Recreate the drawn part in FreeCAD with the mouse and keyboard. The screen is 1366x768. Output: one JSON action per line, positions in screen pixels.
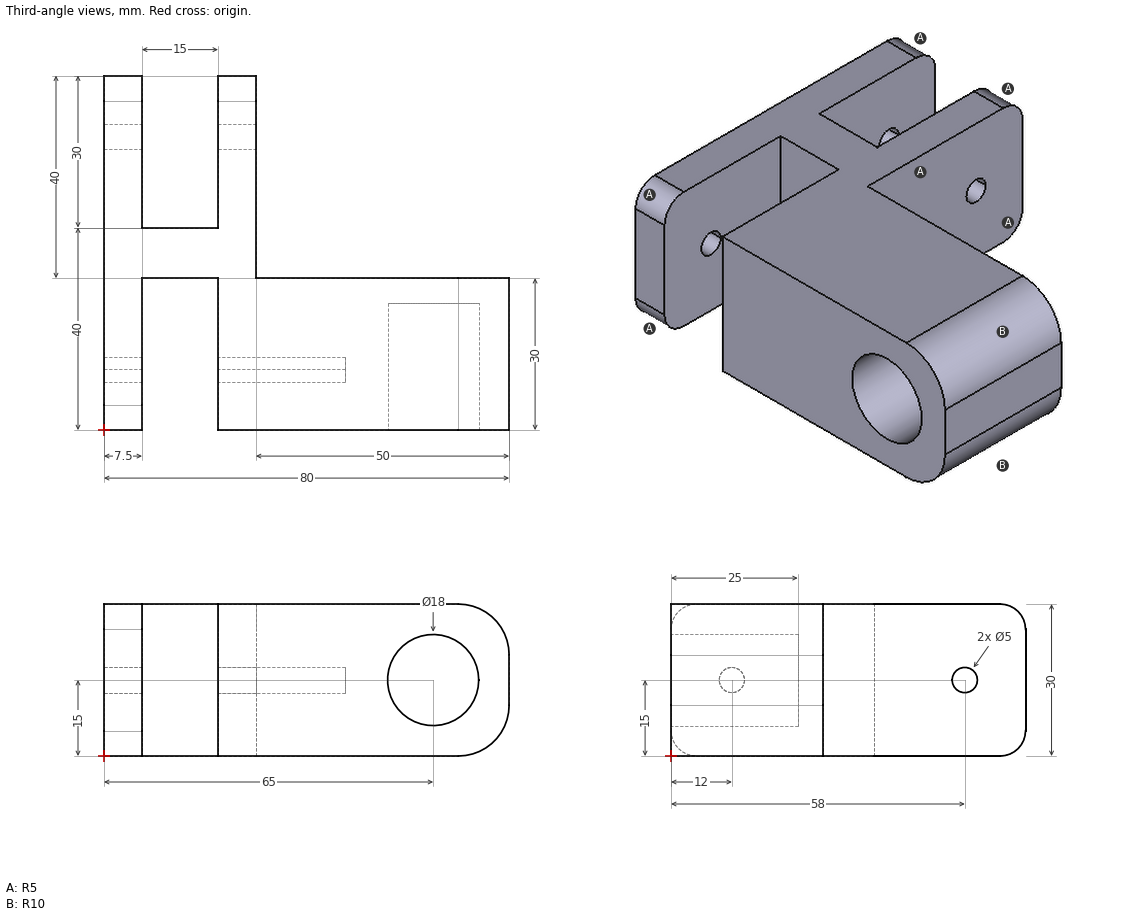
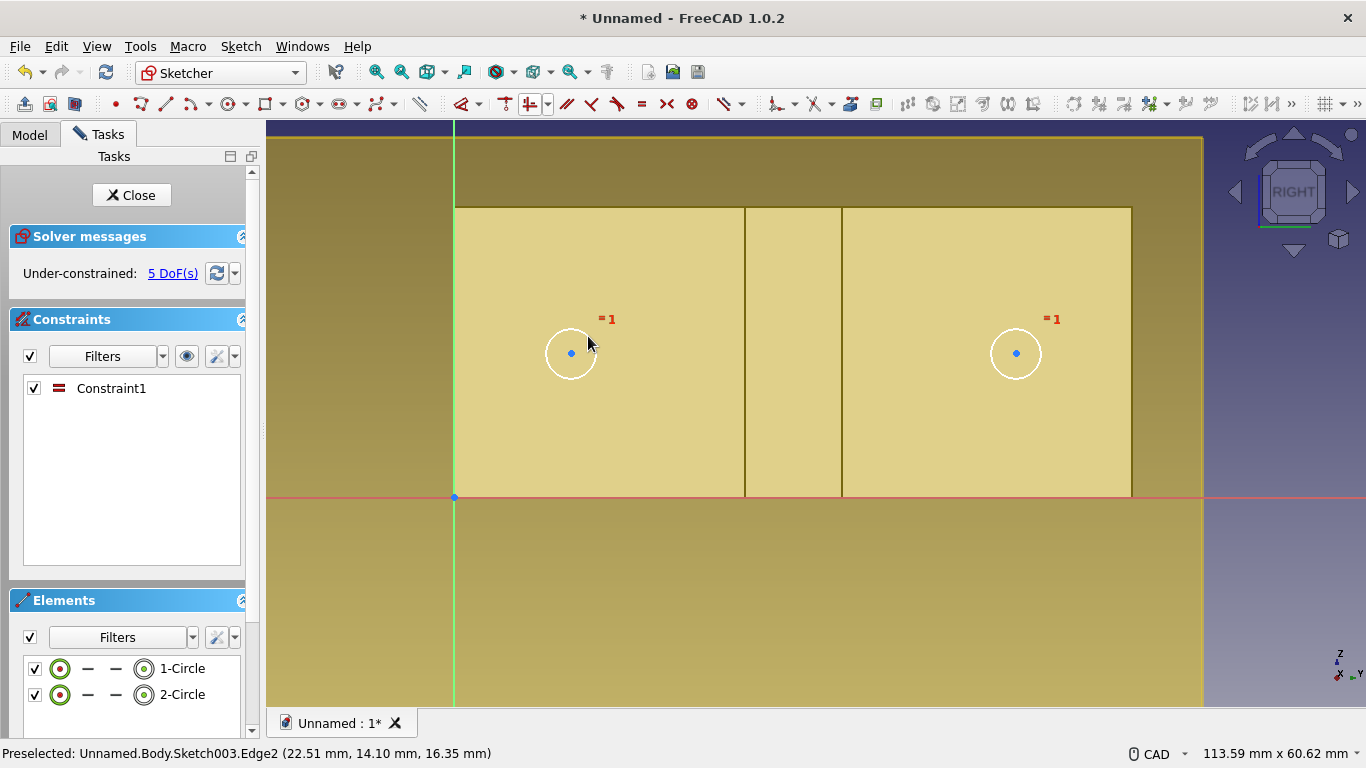
{"action": "left_click", "coordinate": [1016, 354]}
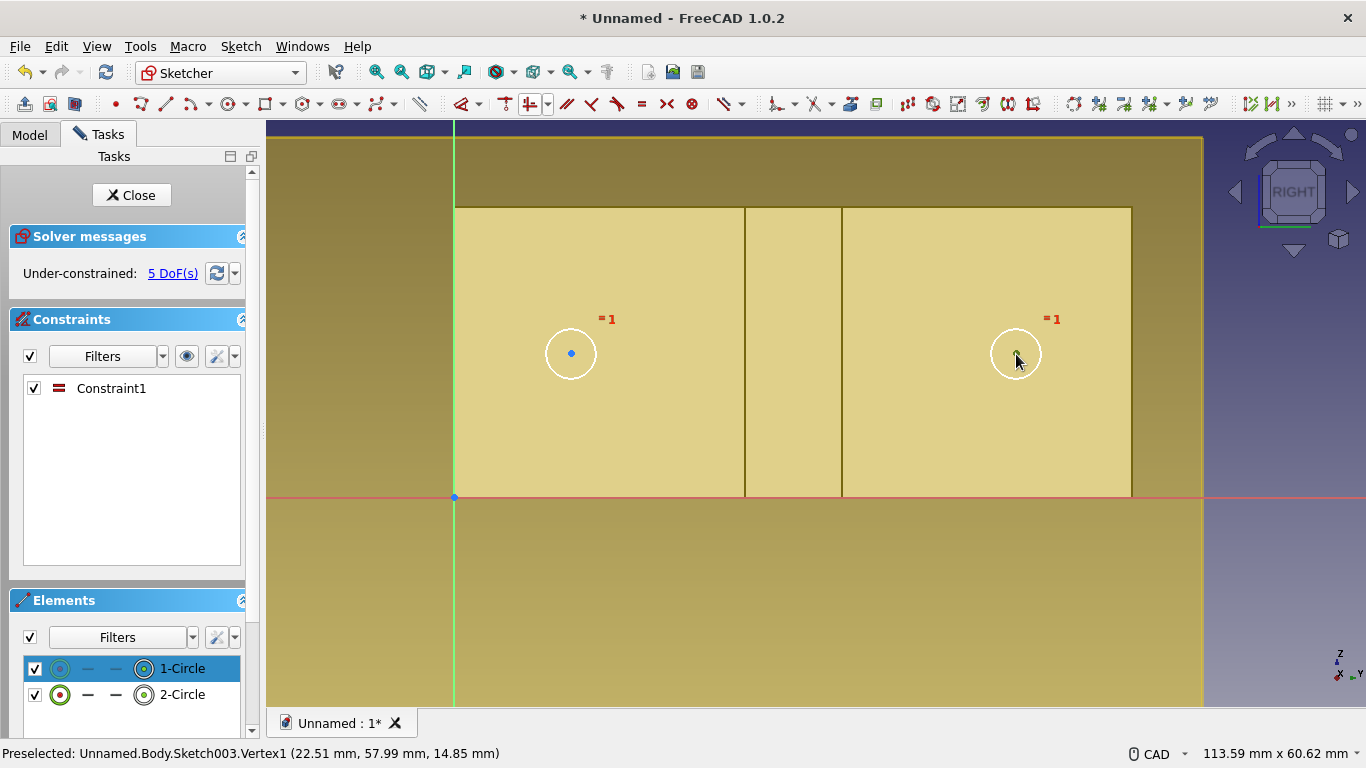
{"action": "left_click", "coordinate": [571, 354]}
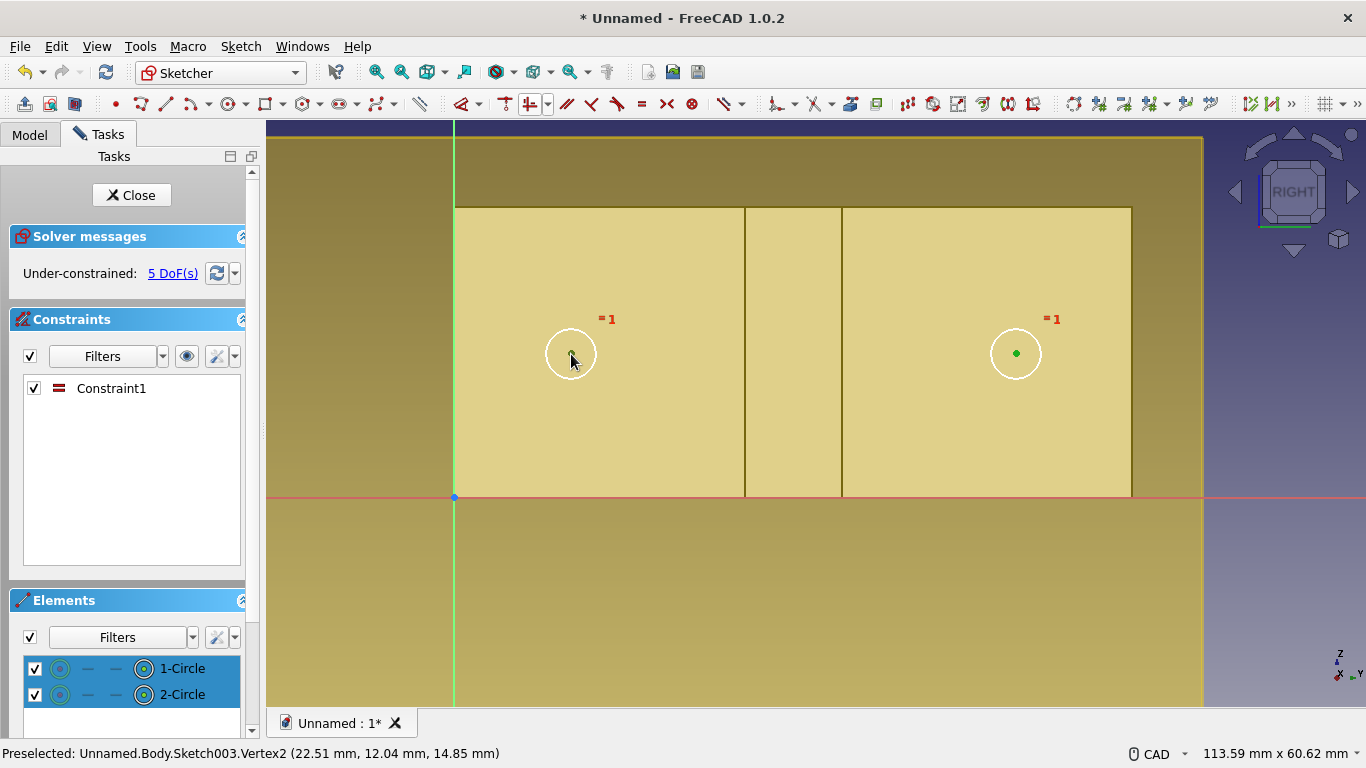
{"action": "key", "text": "h"}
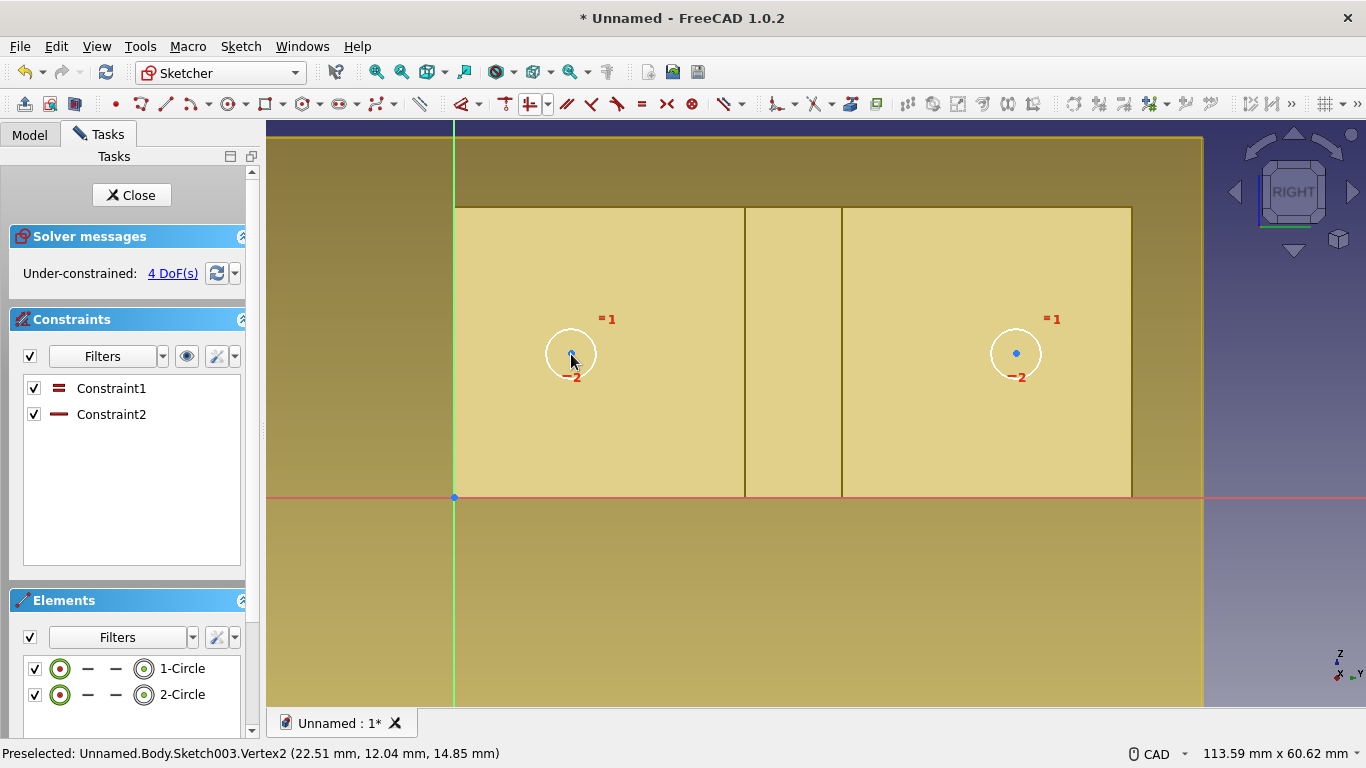
{"action": "left_click", "coordinate": [460, 104]}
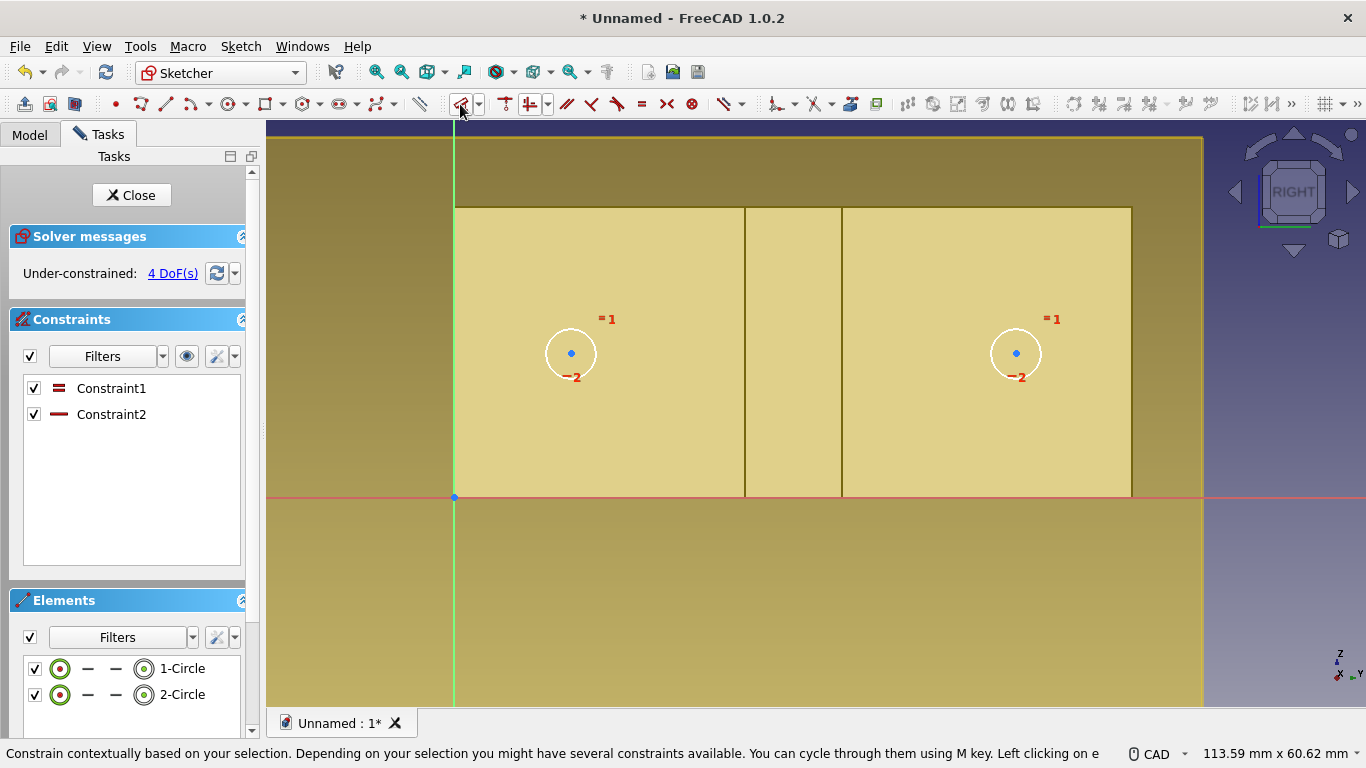
{"action": "left_click", "coordinate": [1033, 336]}
{"action": "left_click", "coordinate": [1055, 313]}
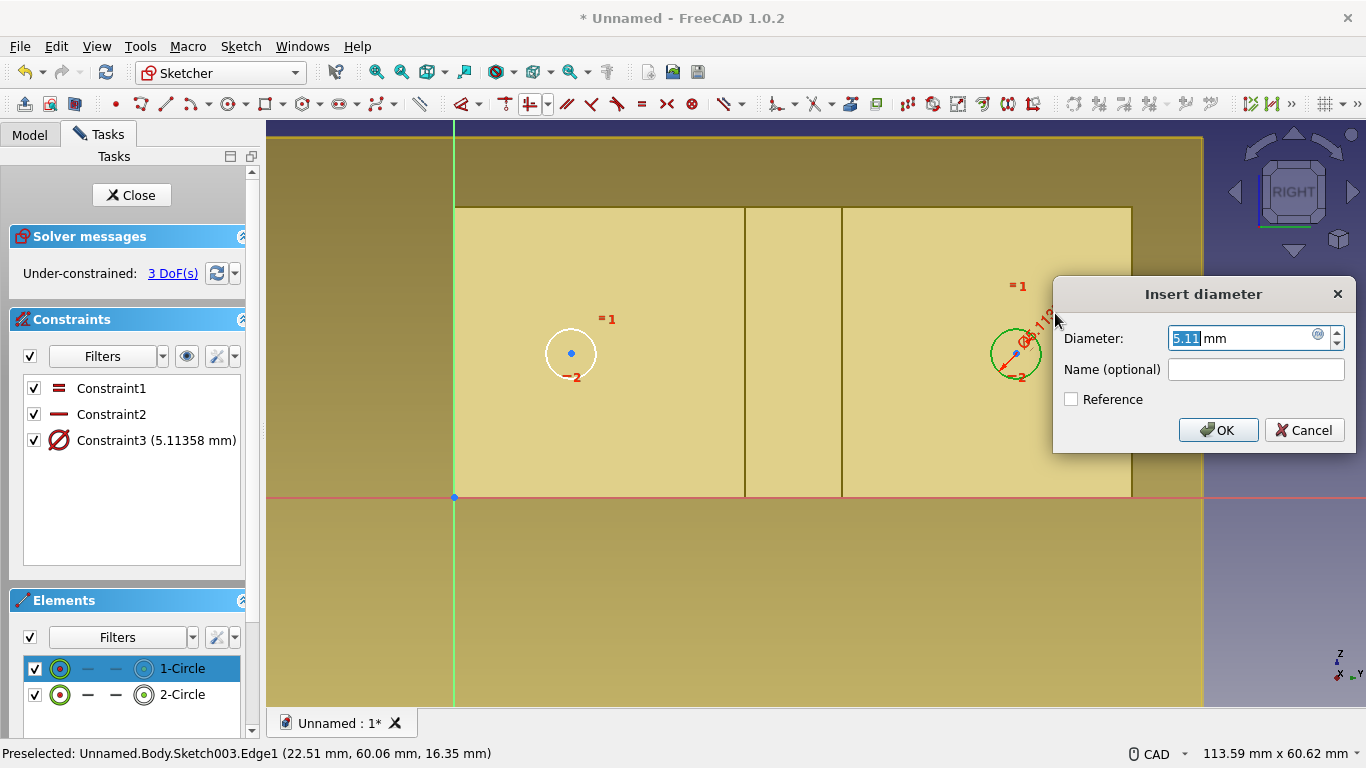
{"action": "type", "text": "5"}
{"action": "key", "text": "Return"}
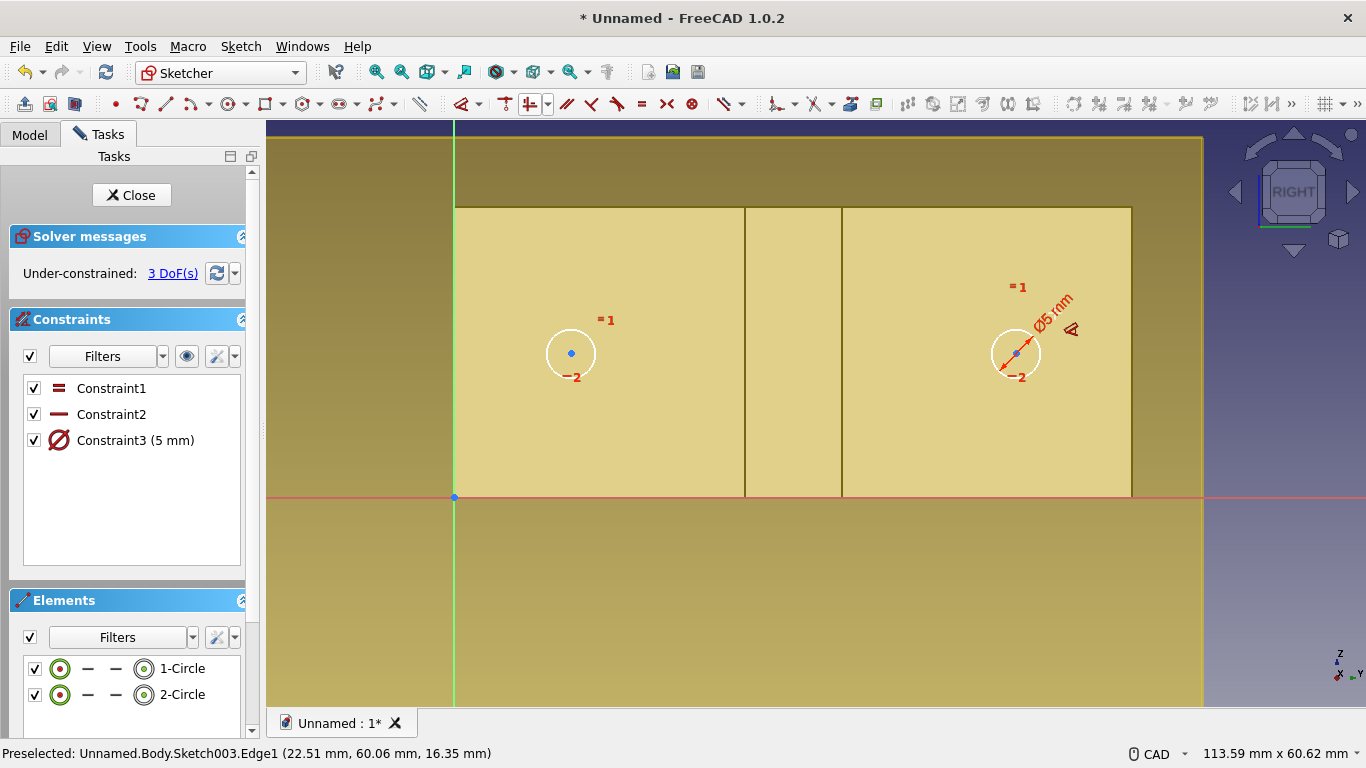
{"action": "left_click", "coordinate": [1016, 354]}
{"action": "left_click", "coordinate": [735, 532]}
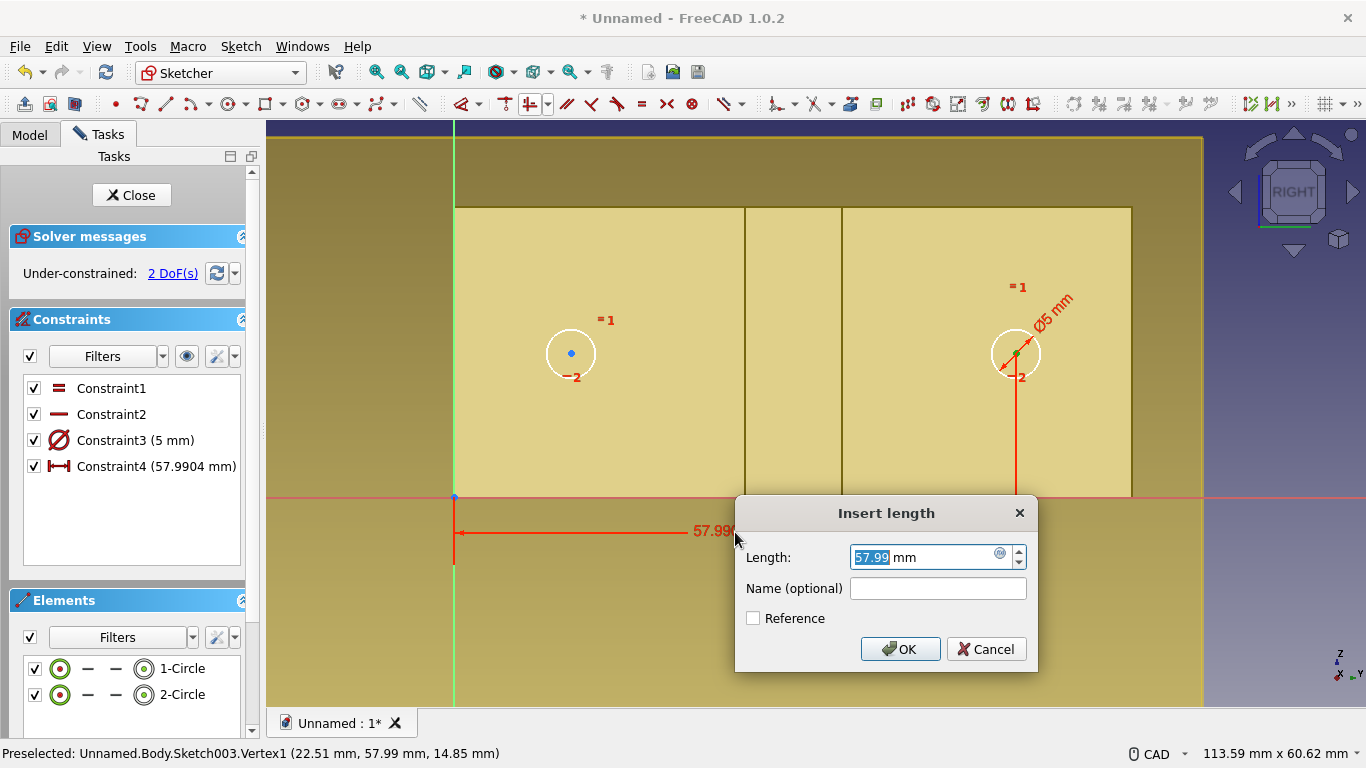
{"action": "type", "text": "58"}
{"action": "key", "text": "Return"}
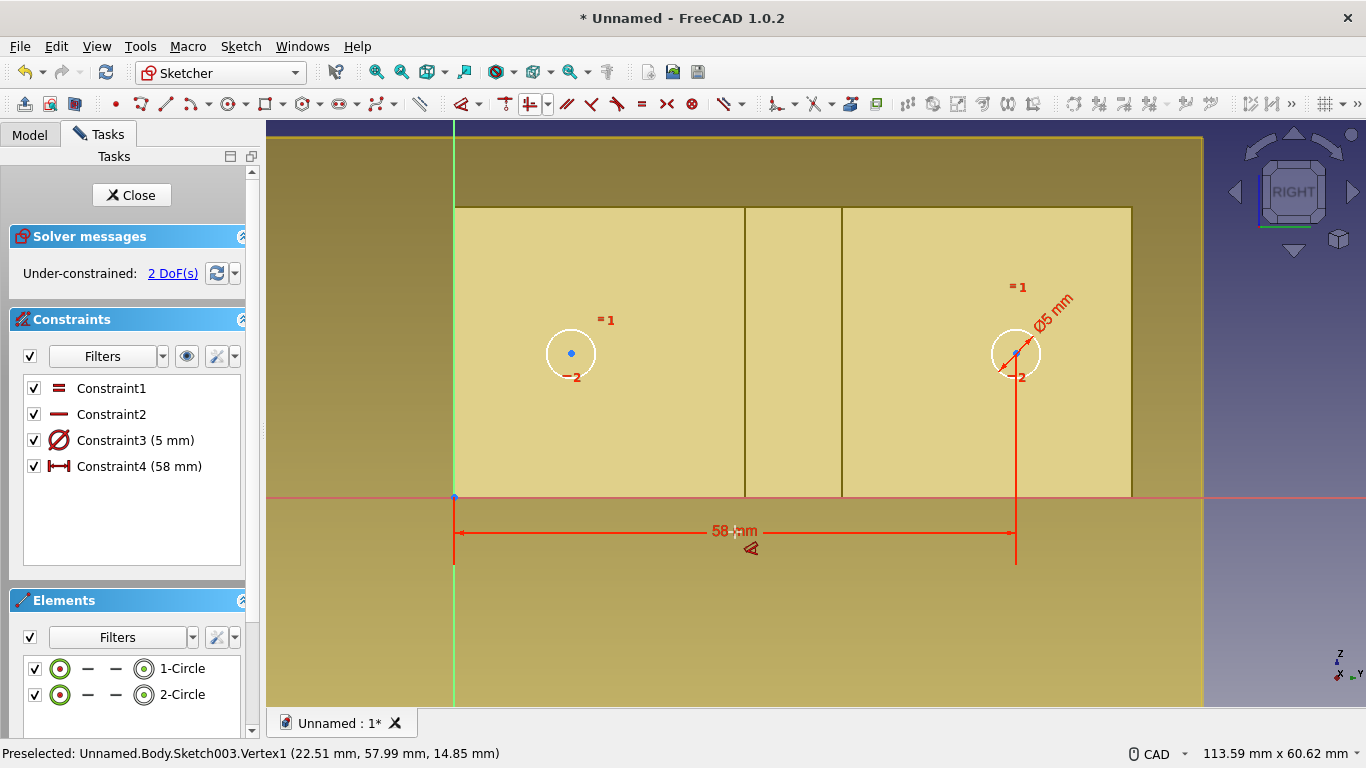
{"action": "left_click", "coordinate": [1016, 354]}
{"action": "left_click", "coordinate": [420, 426]}